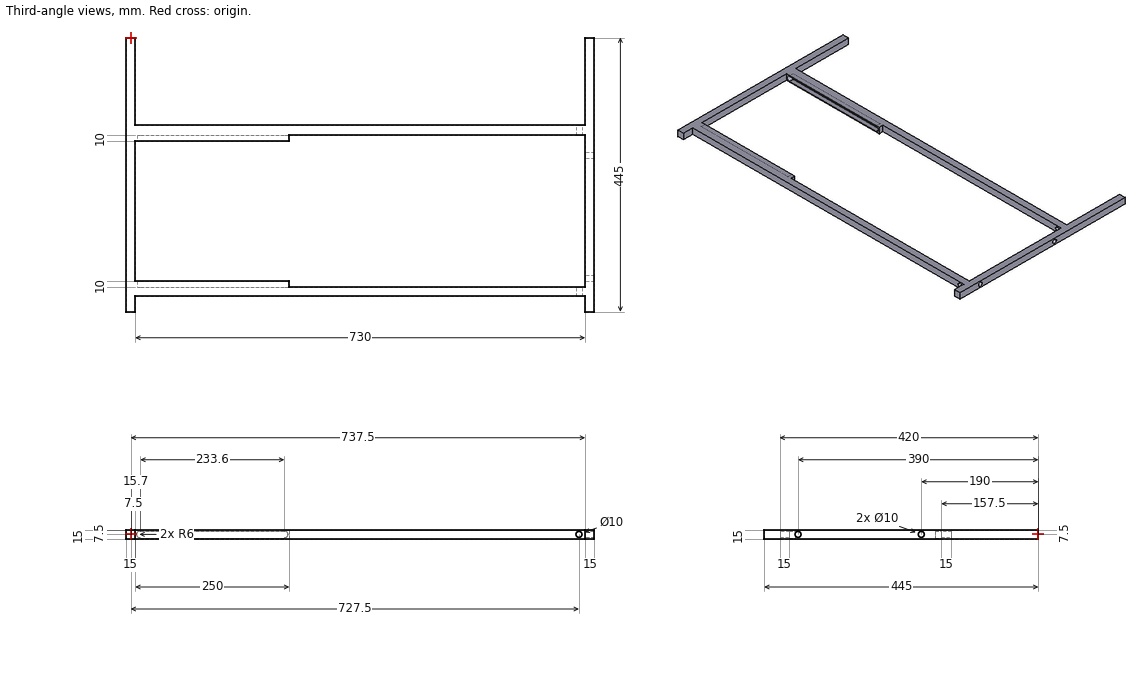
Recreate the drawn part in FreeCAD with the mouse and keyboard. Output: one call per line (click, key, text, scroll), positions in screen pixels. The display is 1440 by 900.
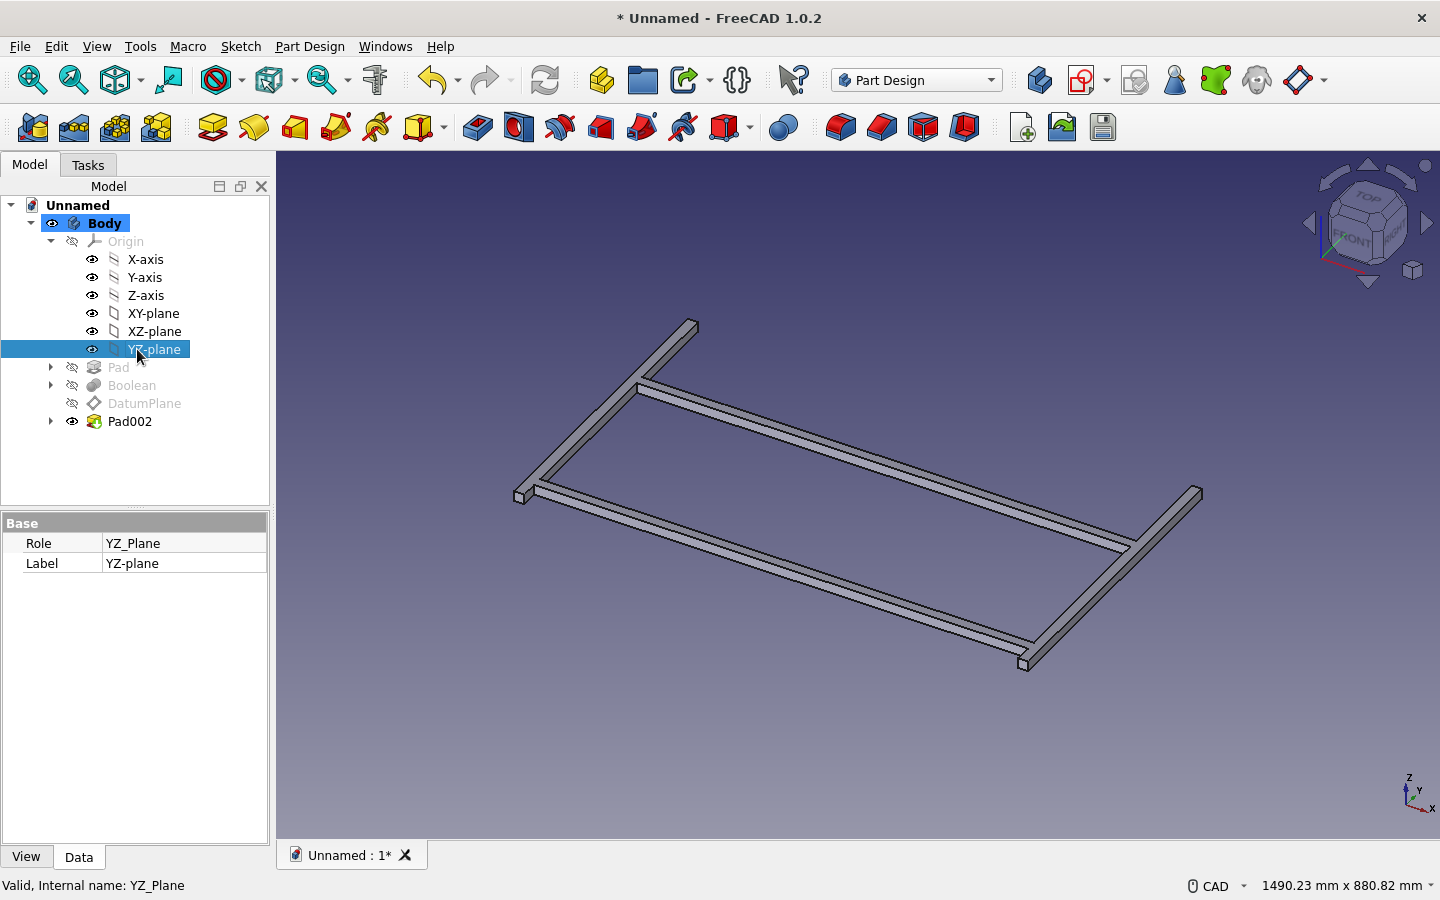
click(1298, 80)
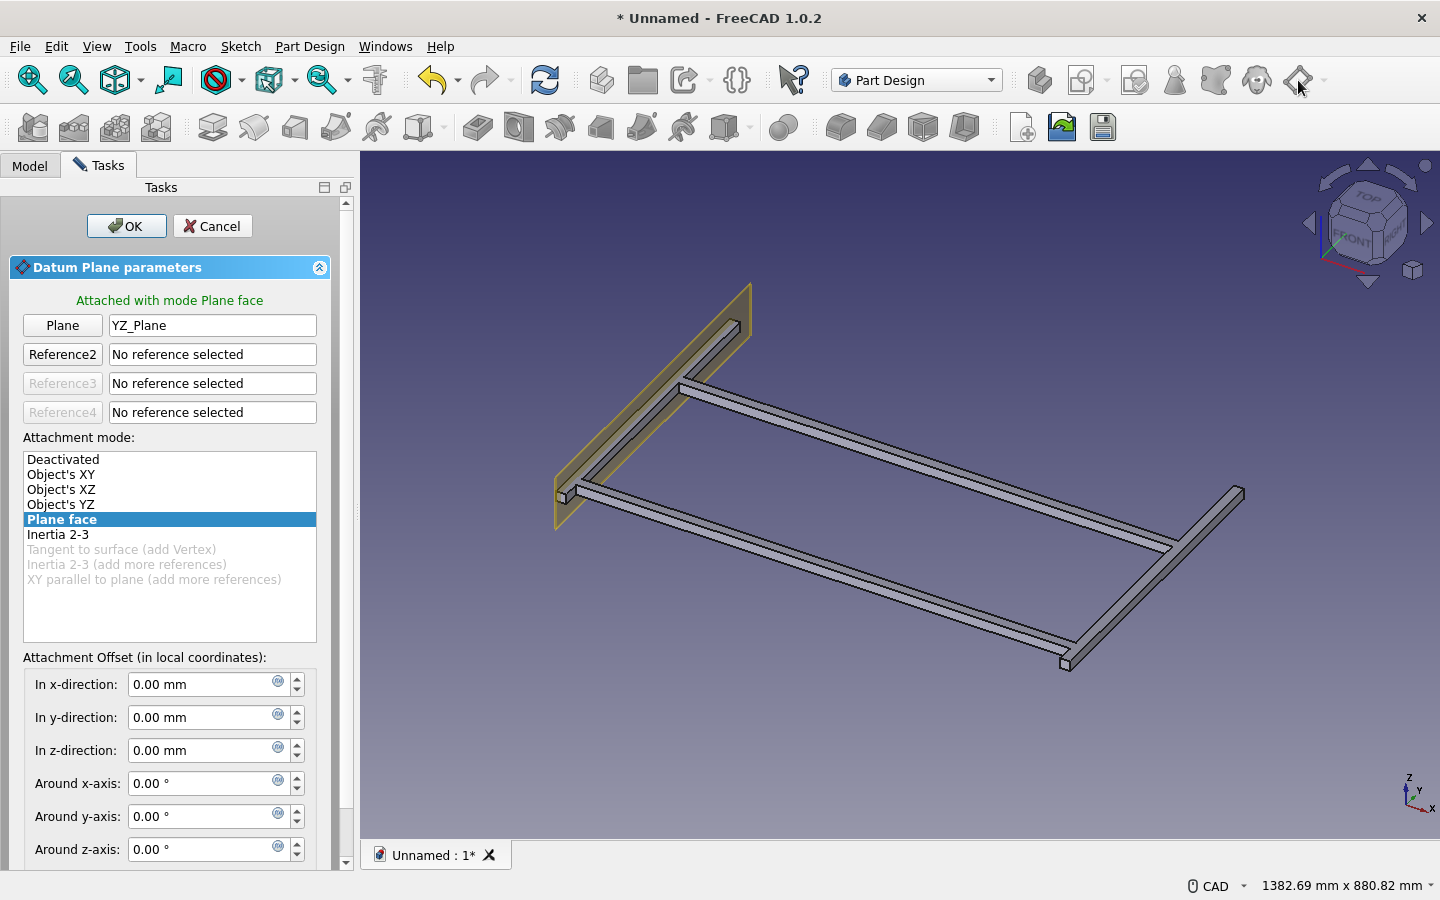
triple_click(210, 750)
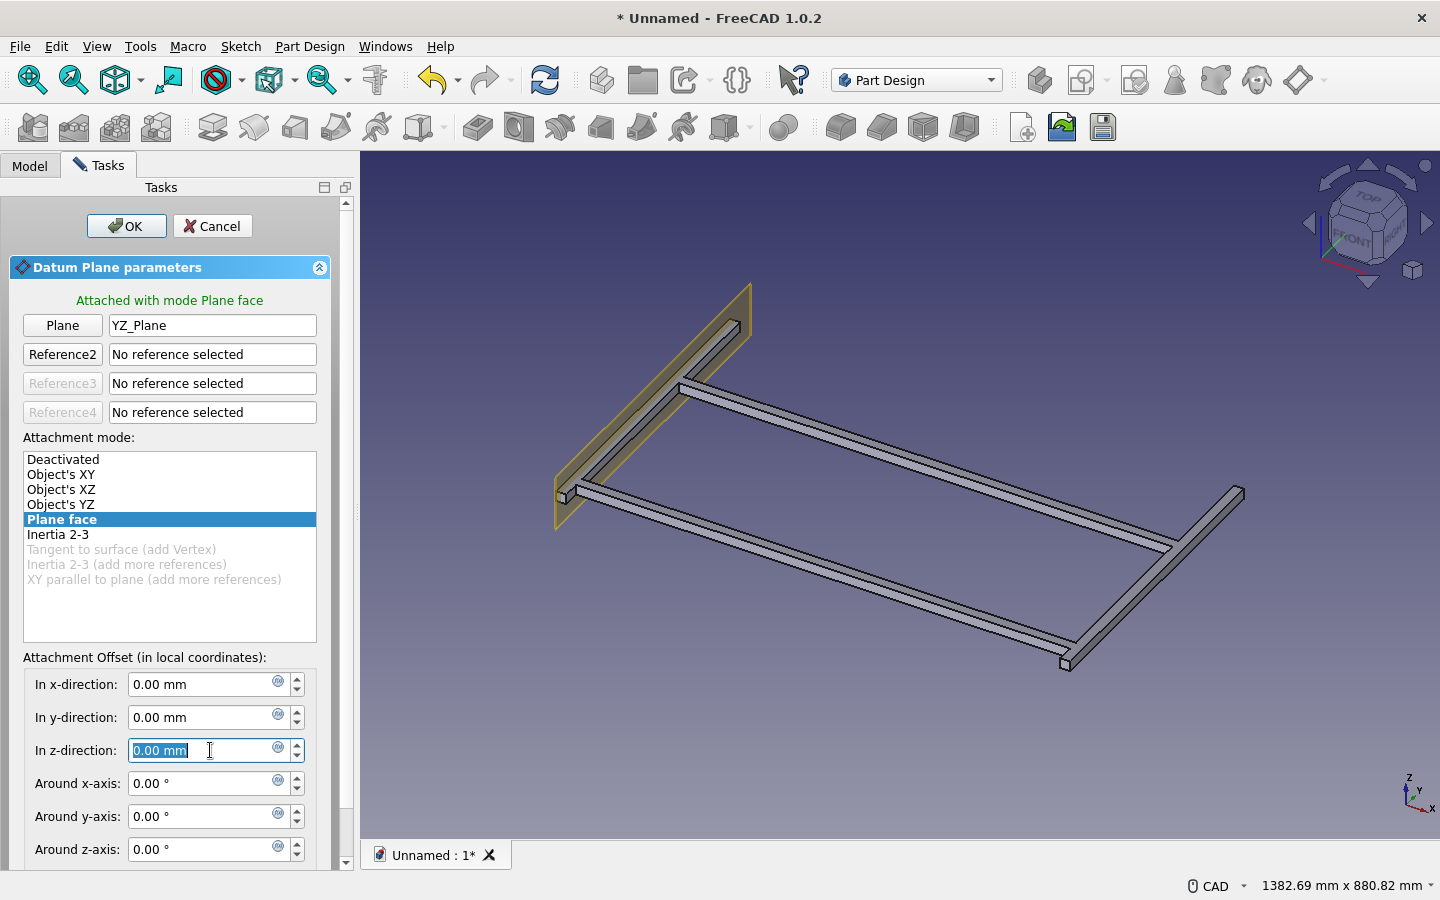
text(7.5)
key(Tab)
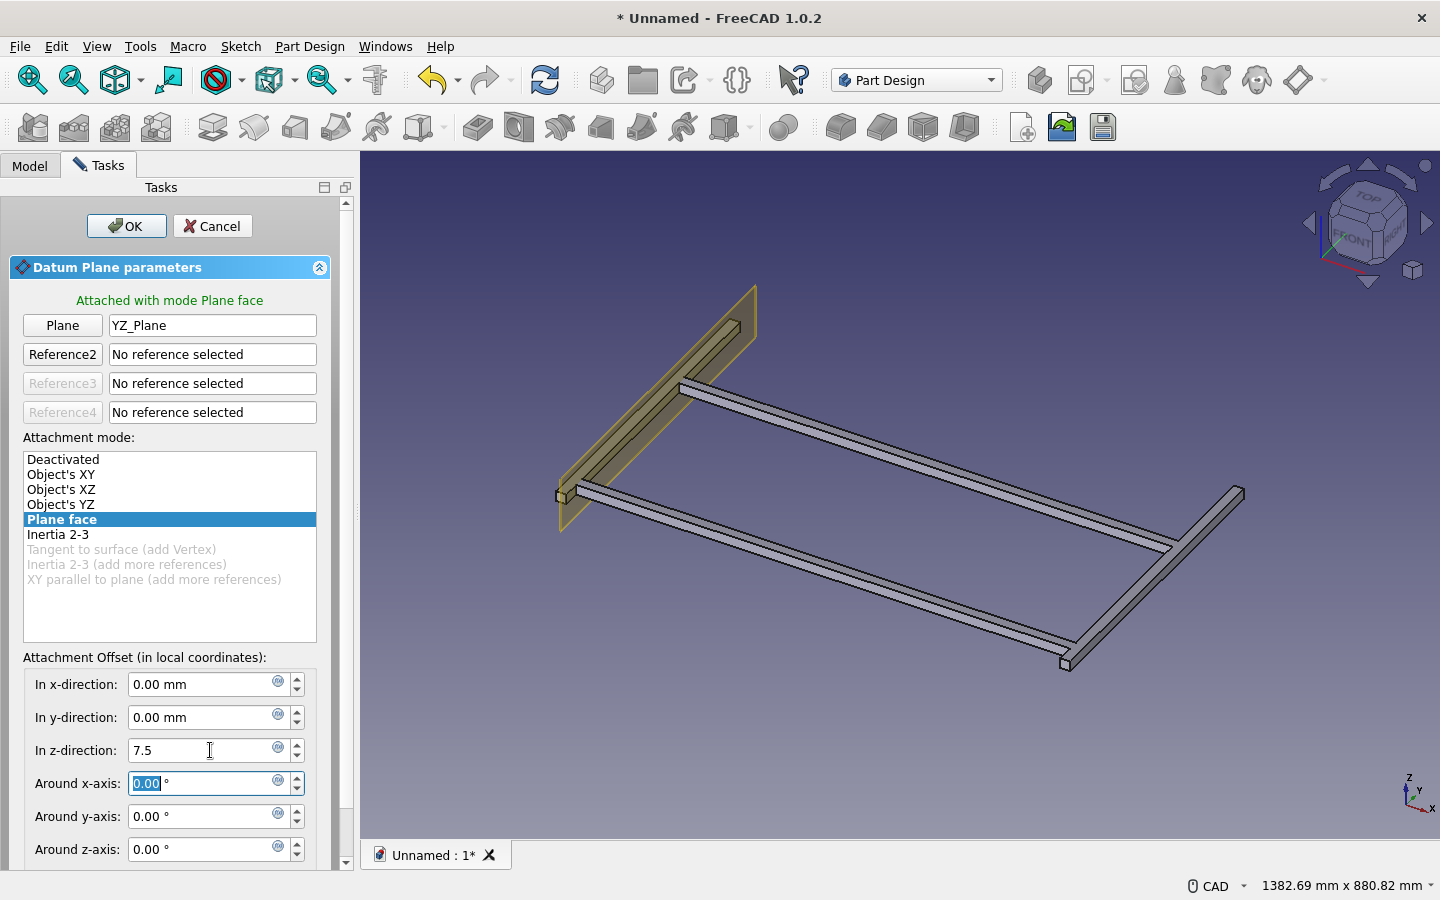
click(127, 226)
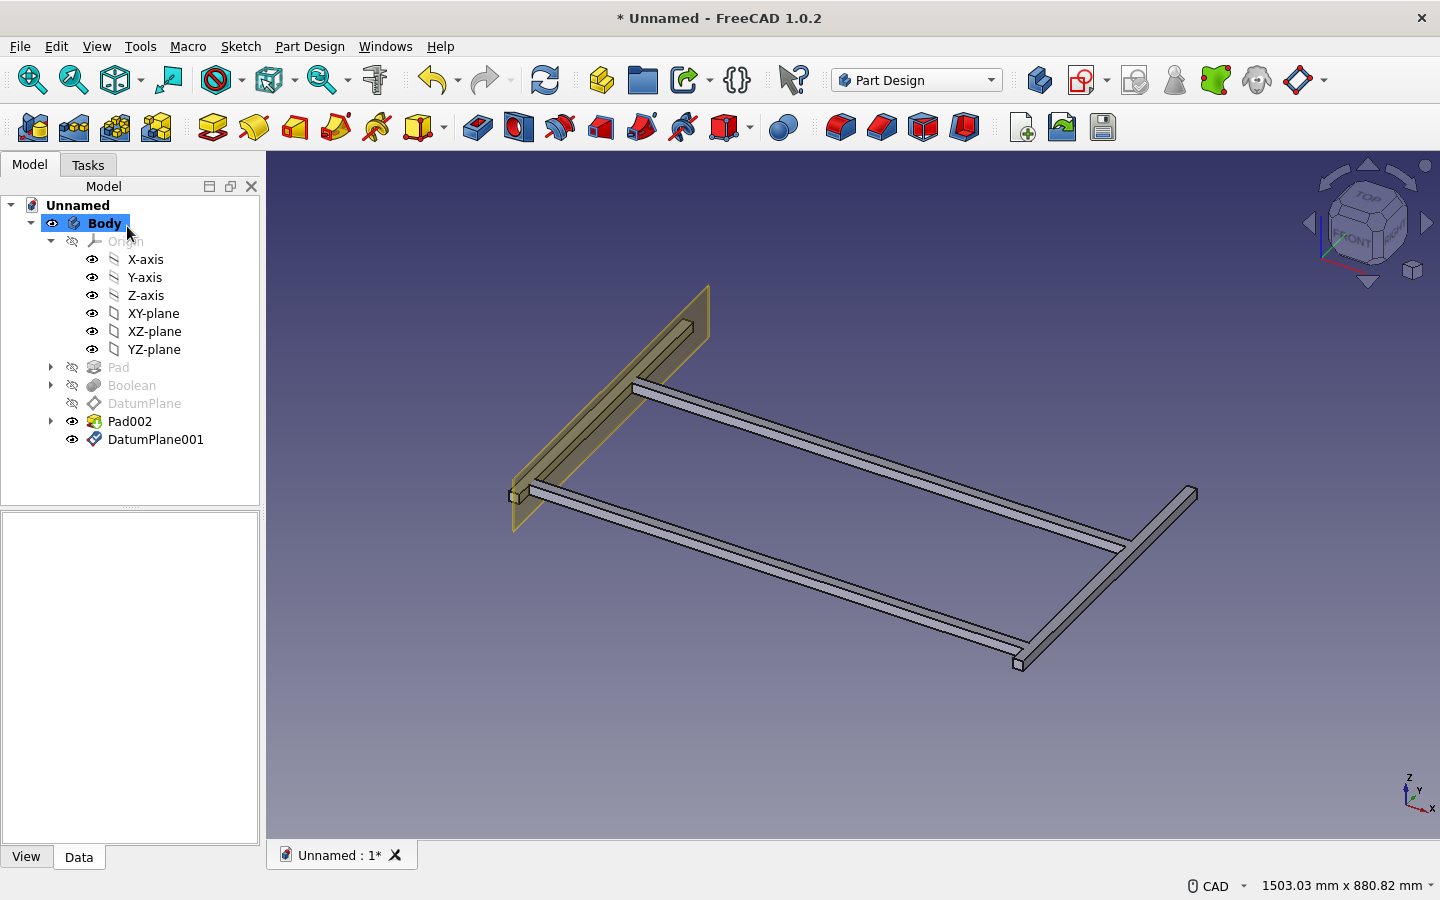
click(117, 439)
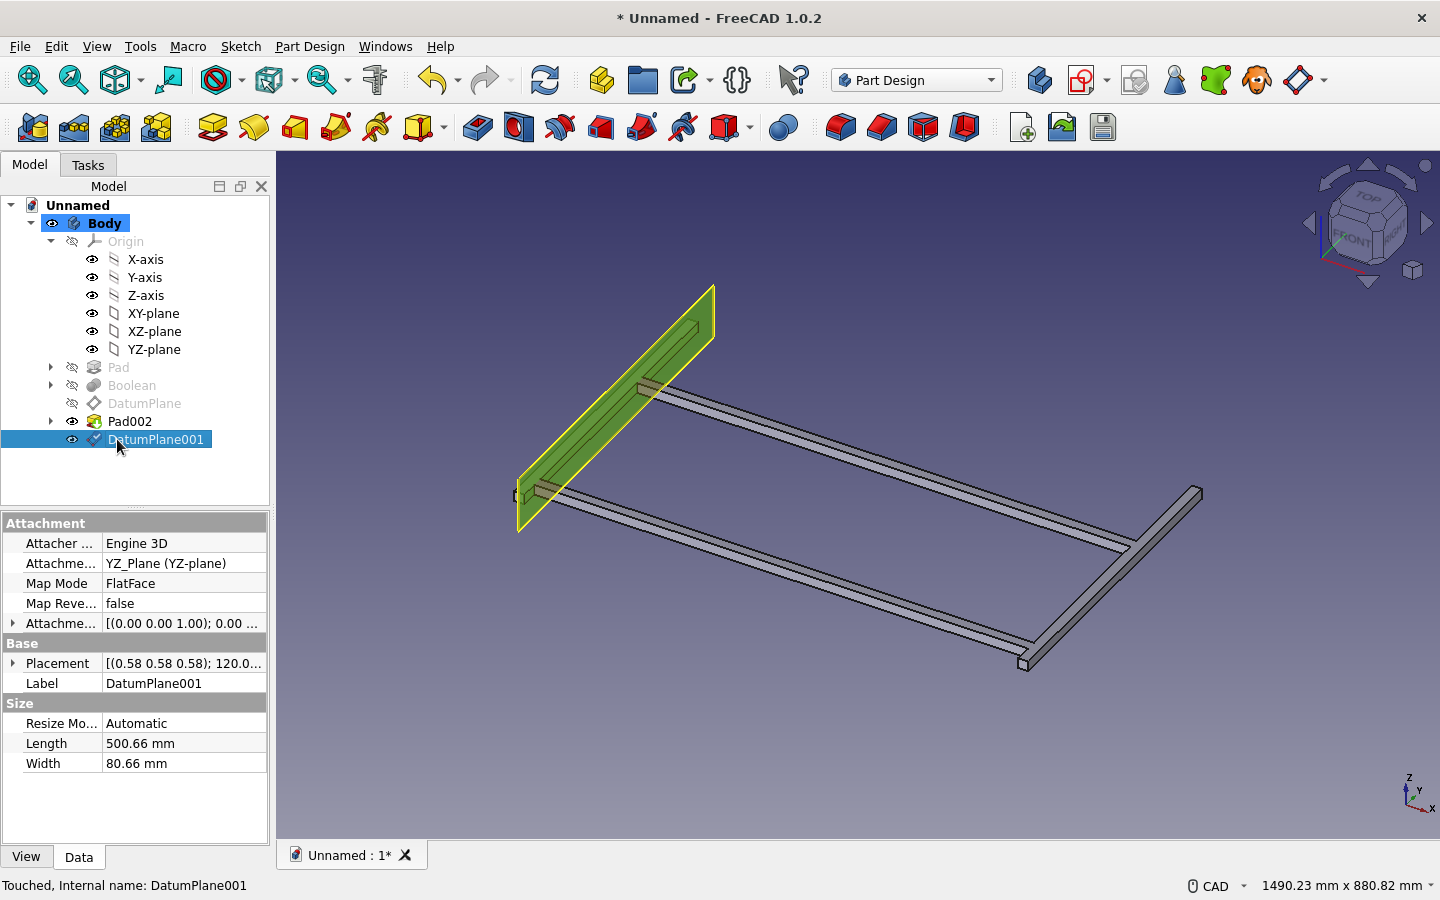
click(1080, 80)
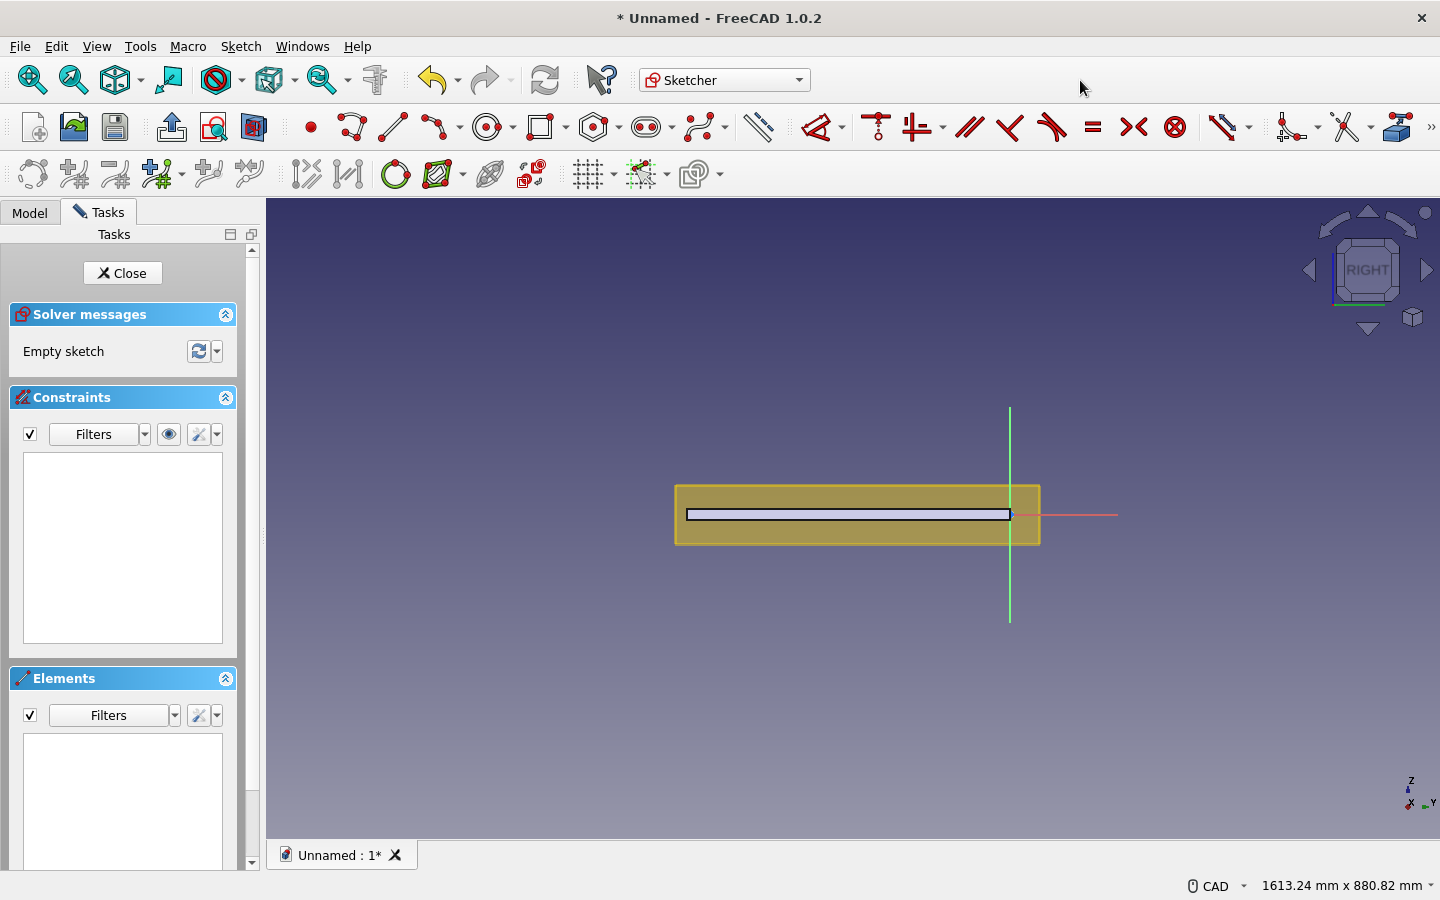
click(254, 128)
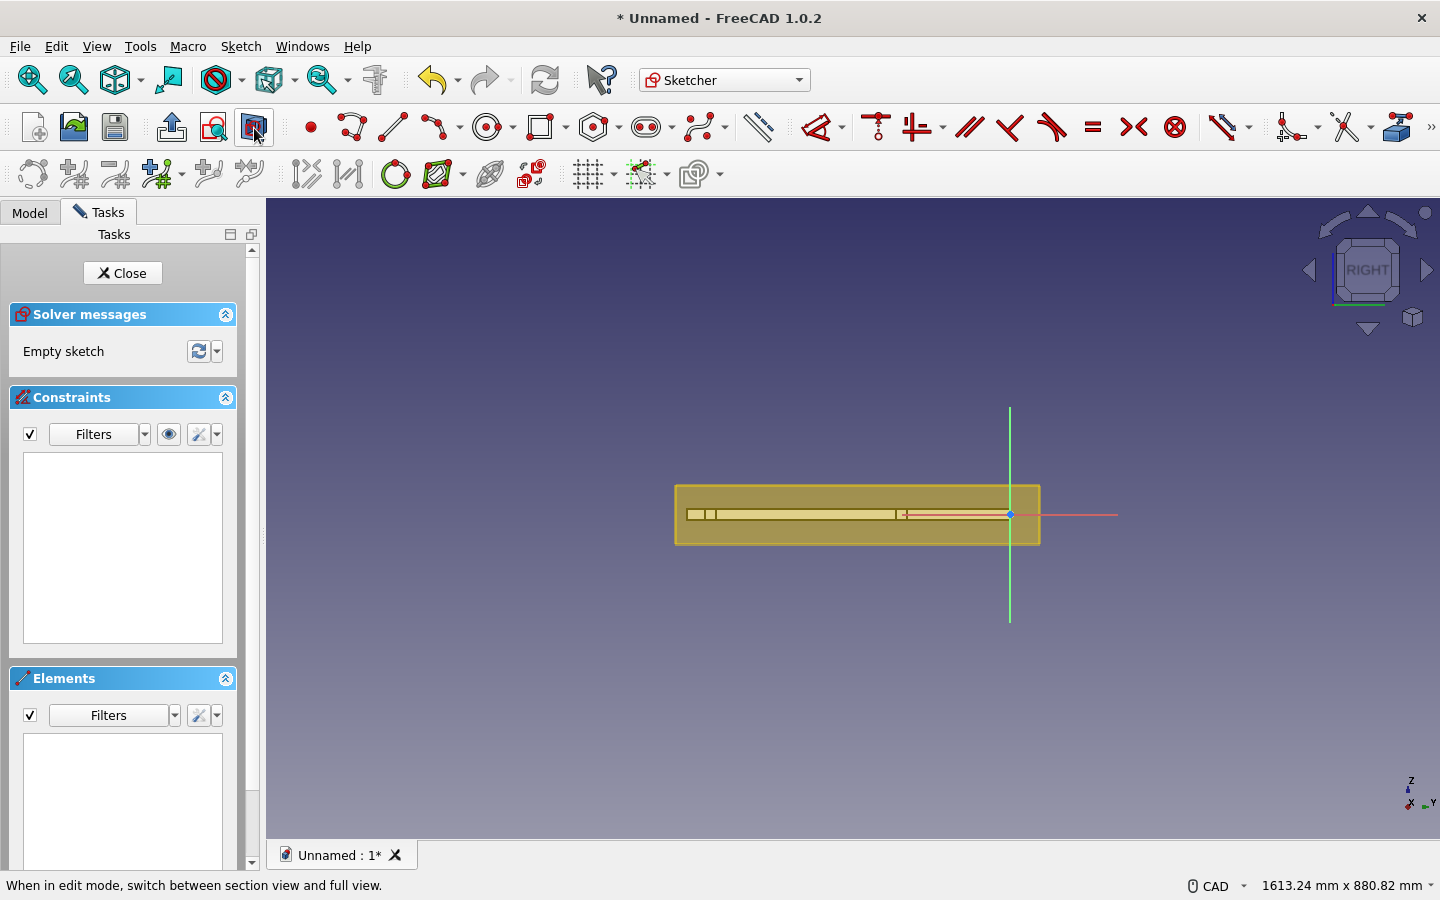
scroll(934, 512, up, 4)